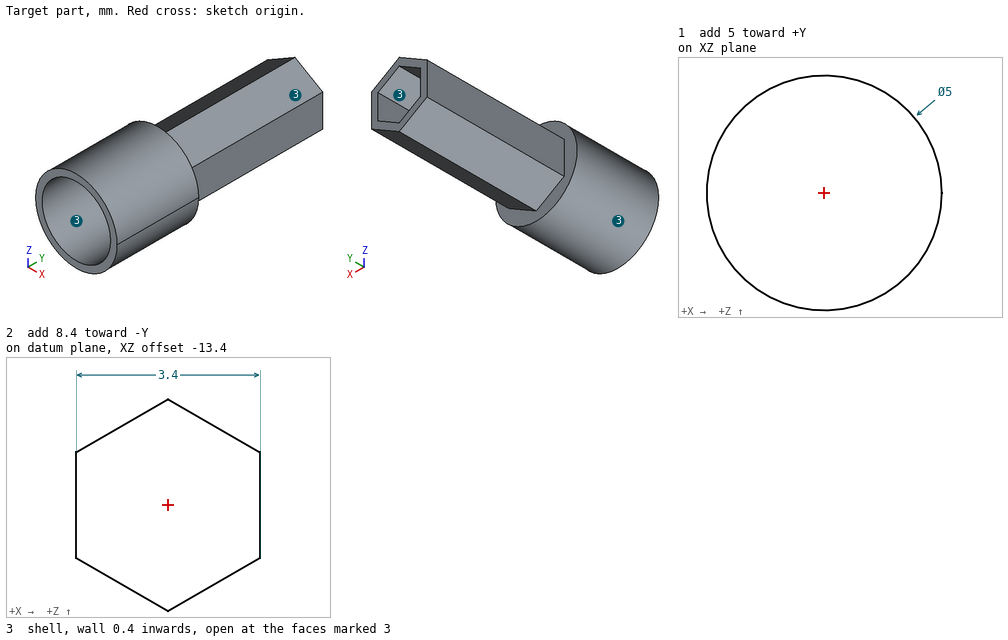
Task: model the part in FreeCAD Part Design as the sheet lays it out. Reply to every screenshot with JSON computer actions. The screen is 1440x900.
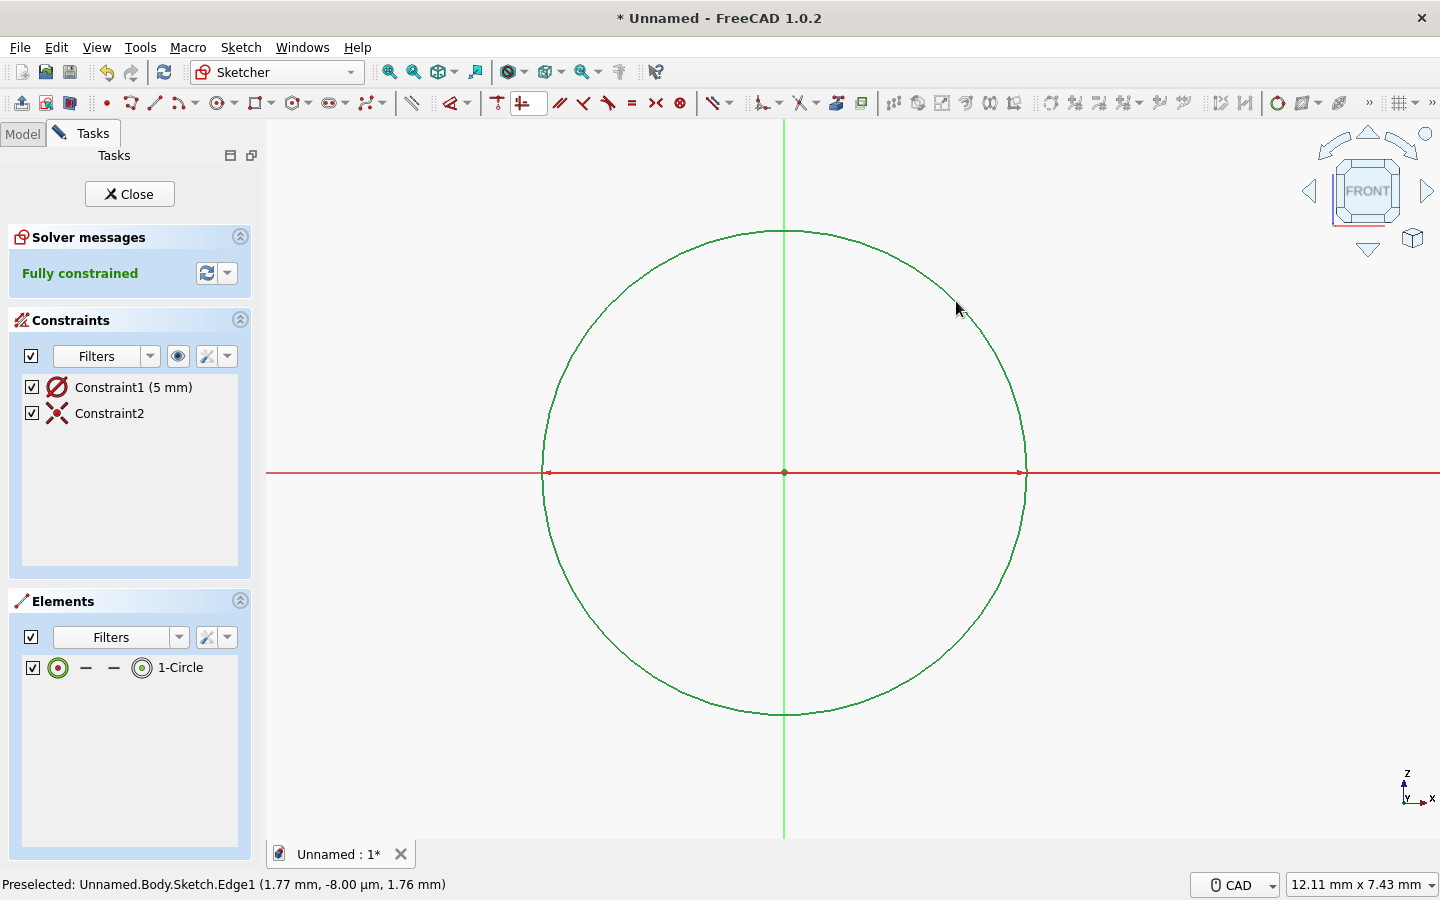
{"action": "left_click", "coordinate": [130, 194]}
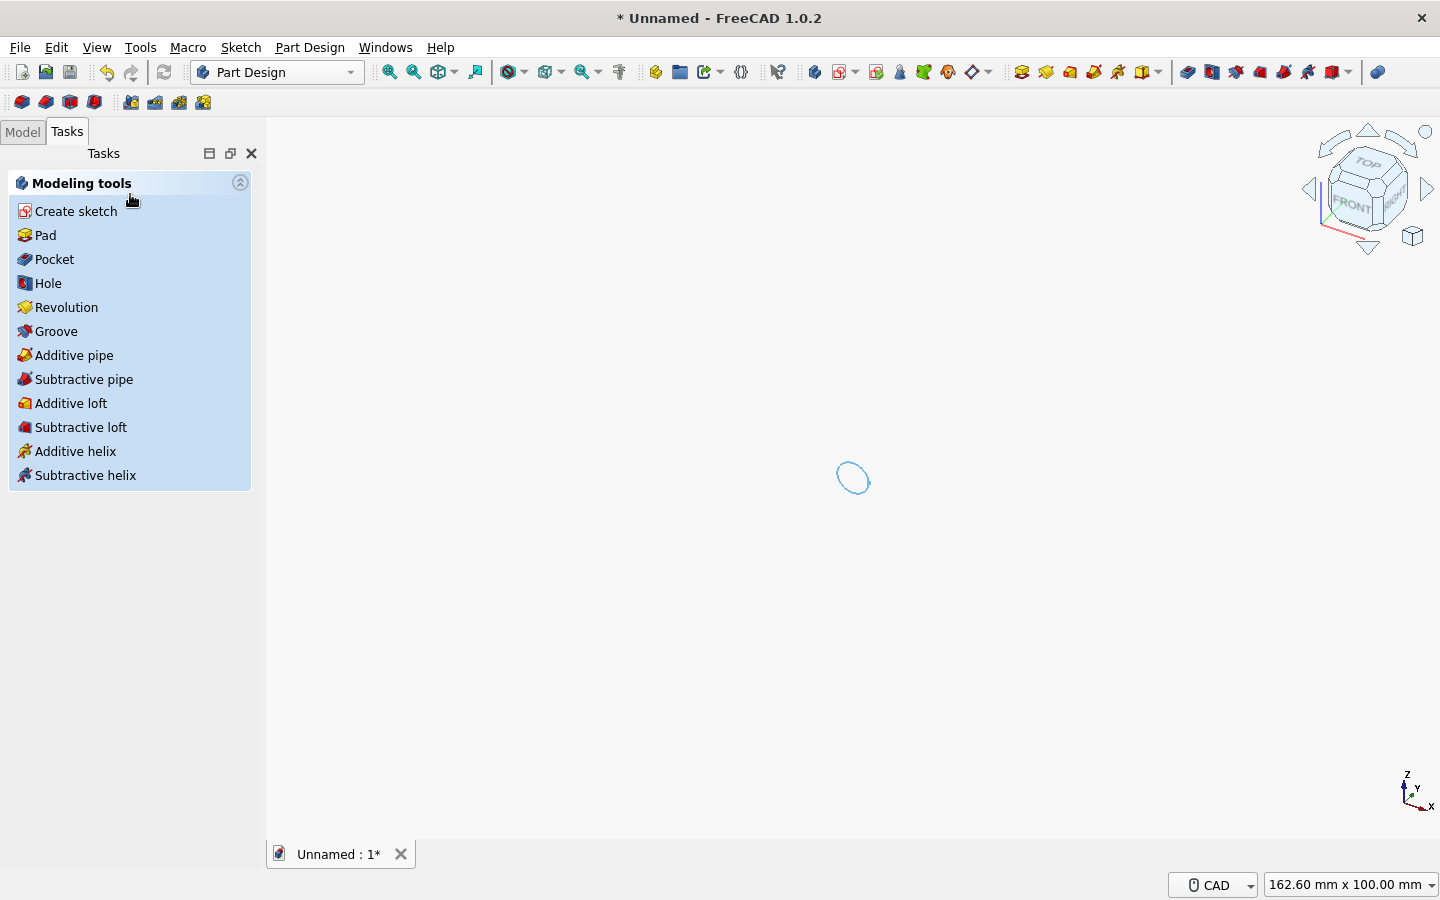
{"action": "left_click", "coordinate": [1022, 72]}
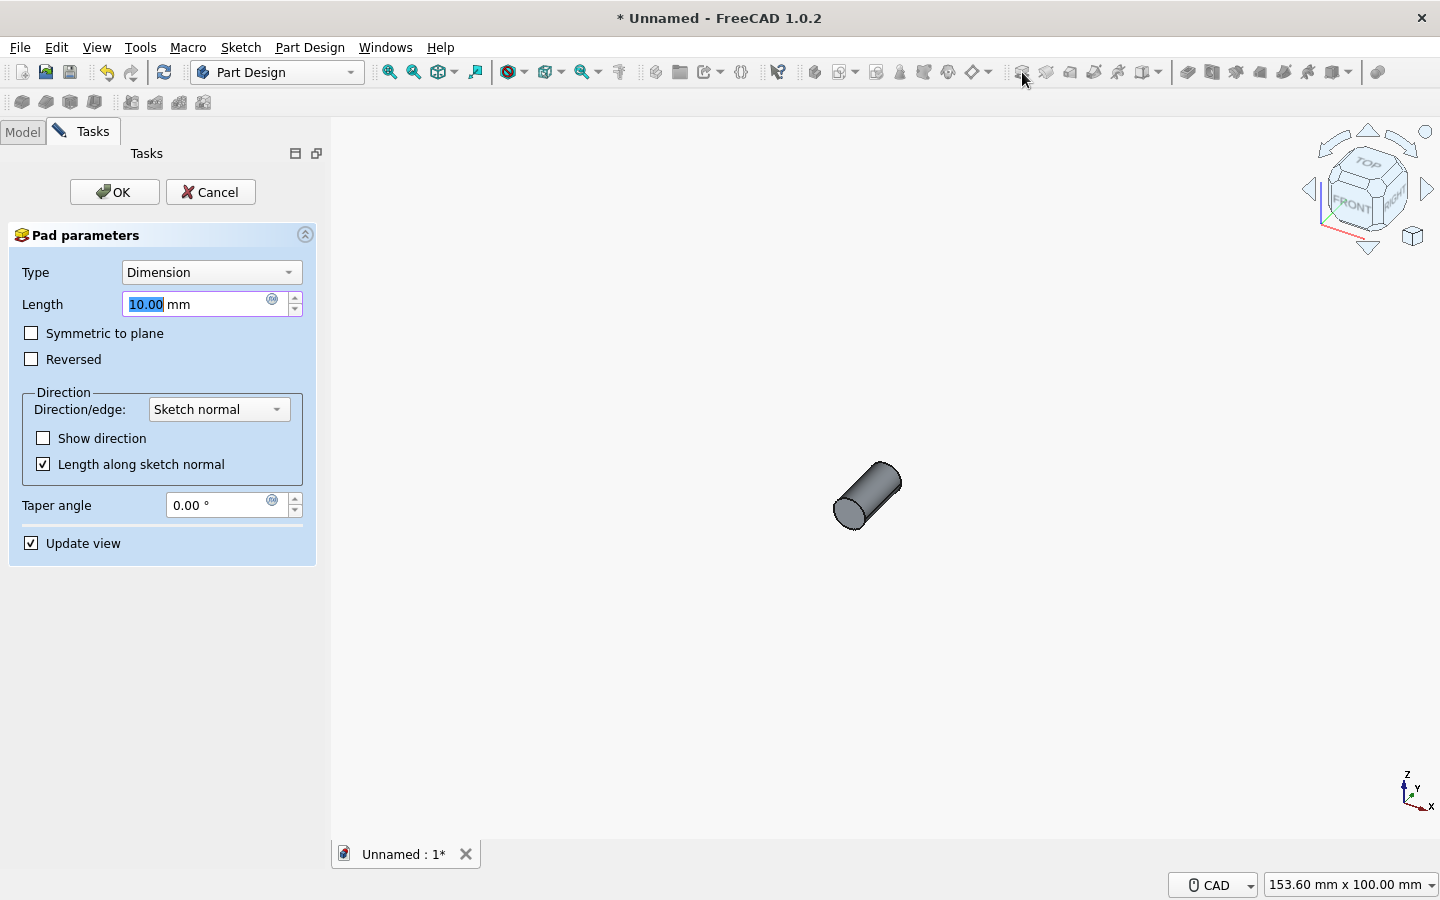
{"action": "type", "text": "5"}
{"action": "key", "text": "Tab"}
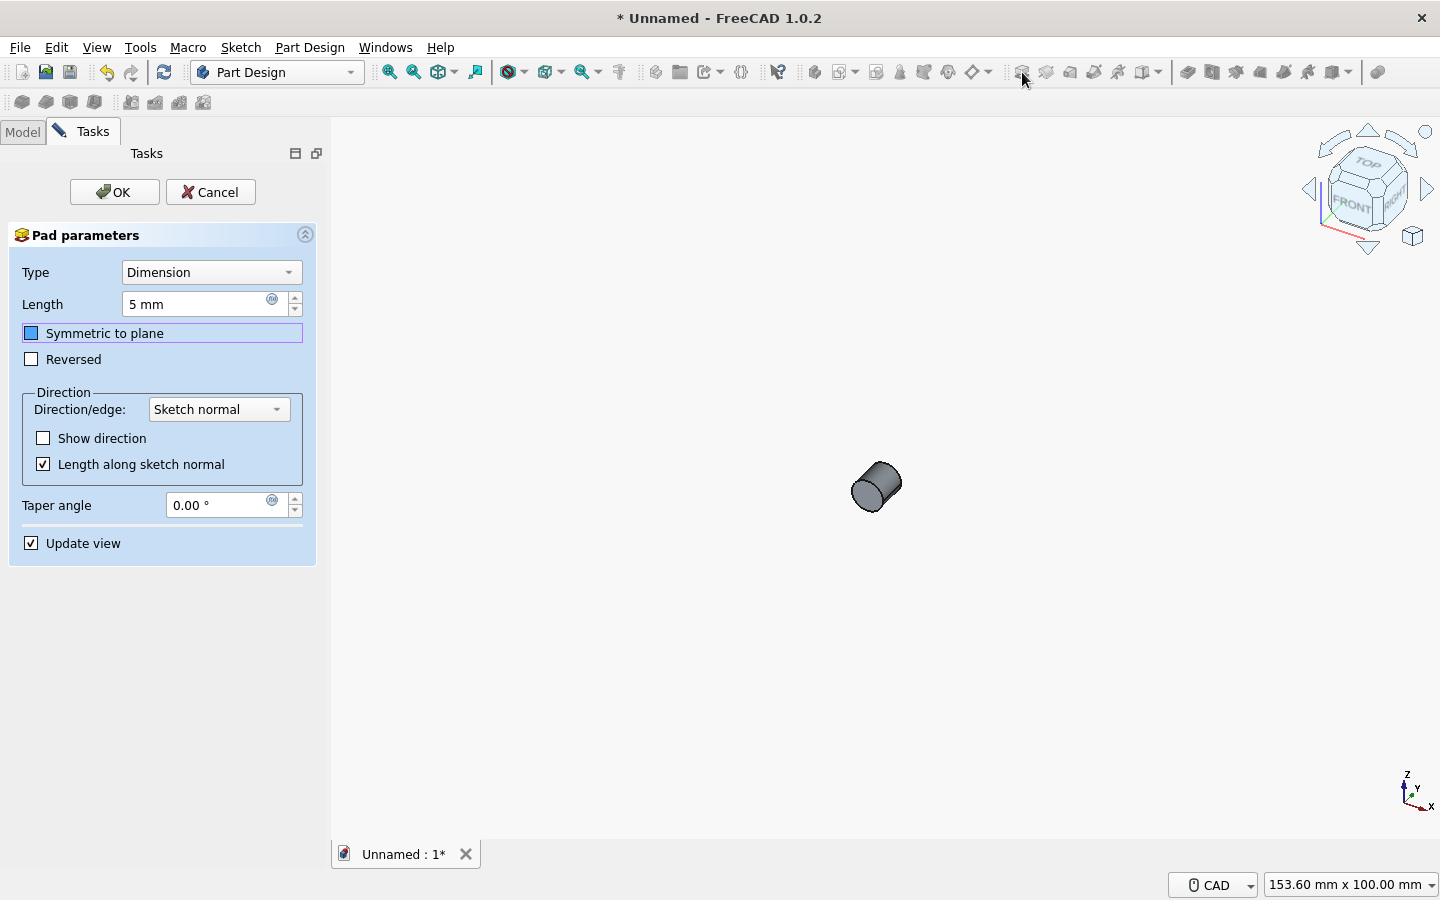
{"action": "left_click", "coordinate": [30, 359]}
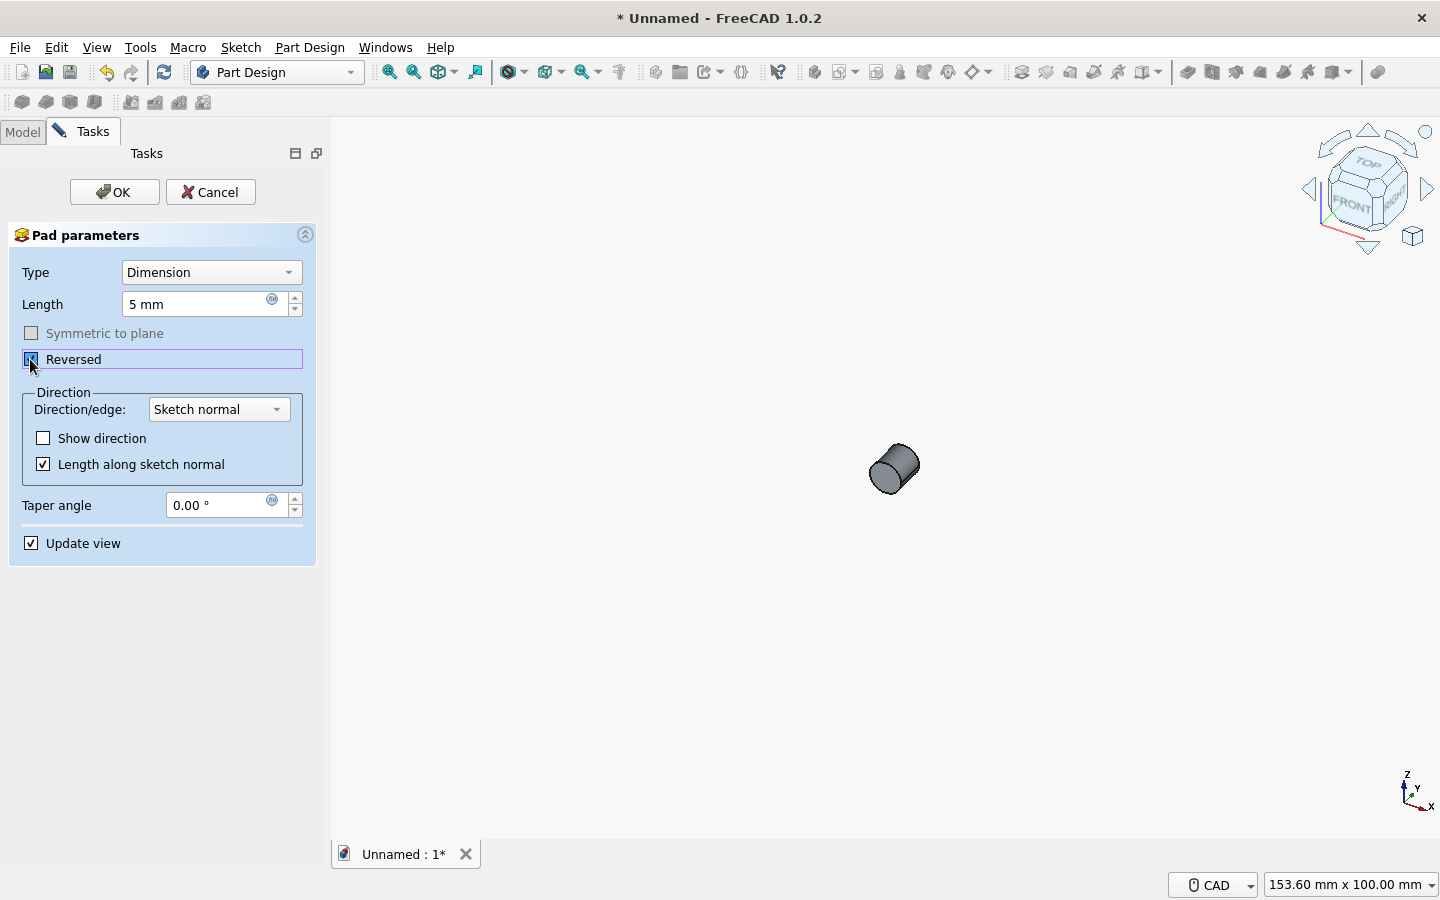
{"action": "left_click", "coordinate": [115, 192]}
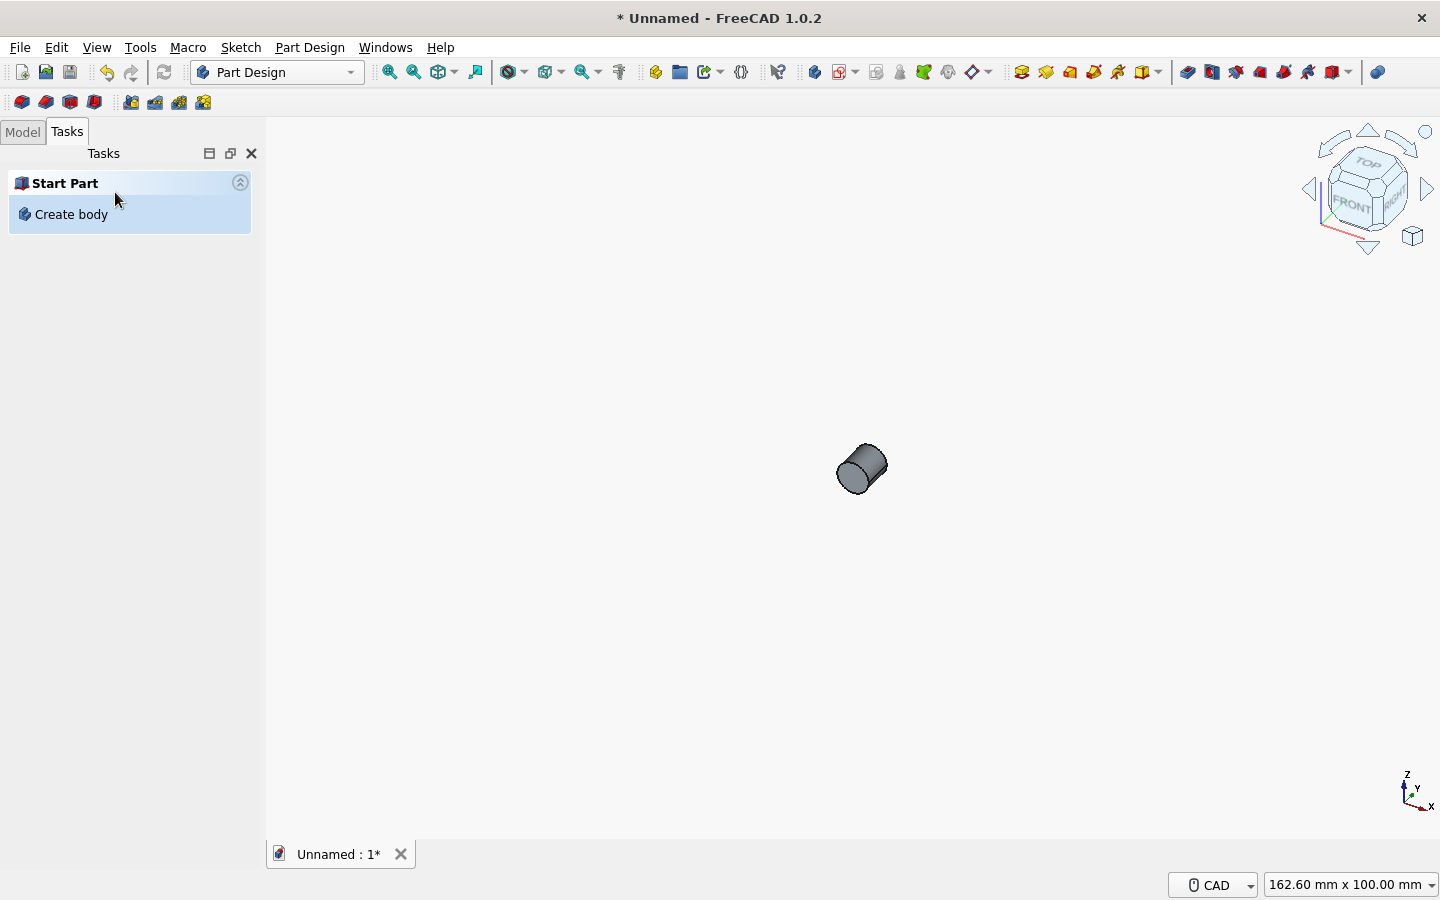
{"action": "left_click", "coordinate": [390, 72]}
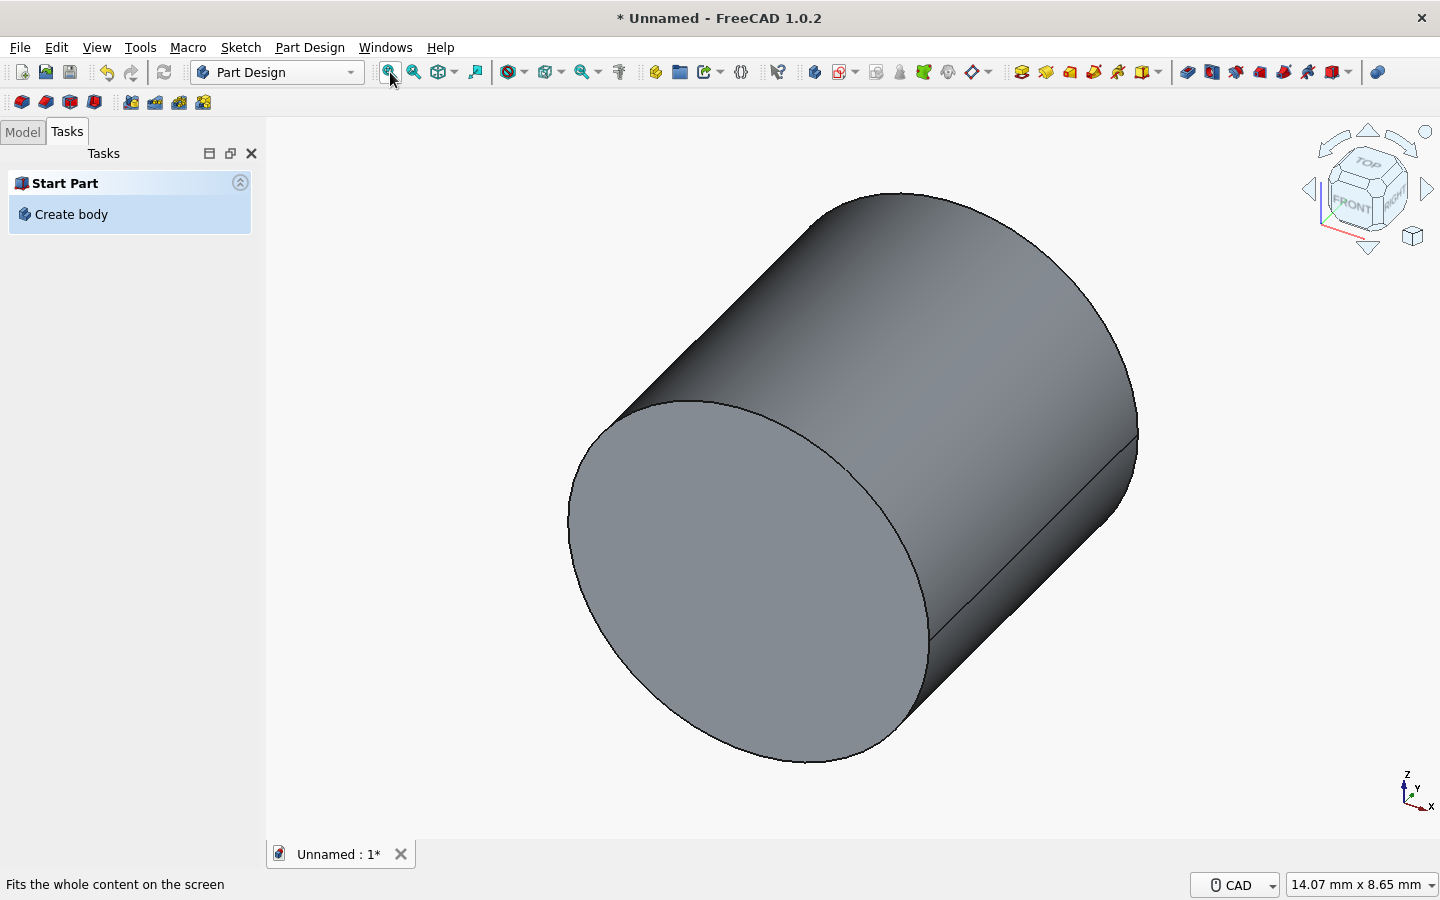
{"action": "left_click", "coordinate": [23, 131]}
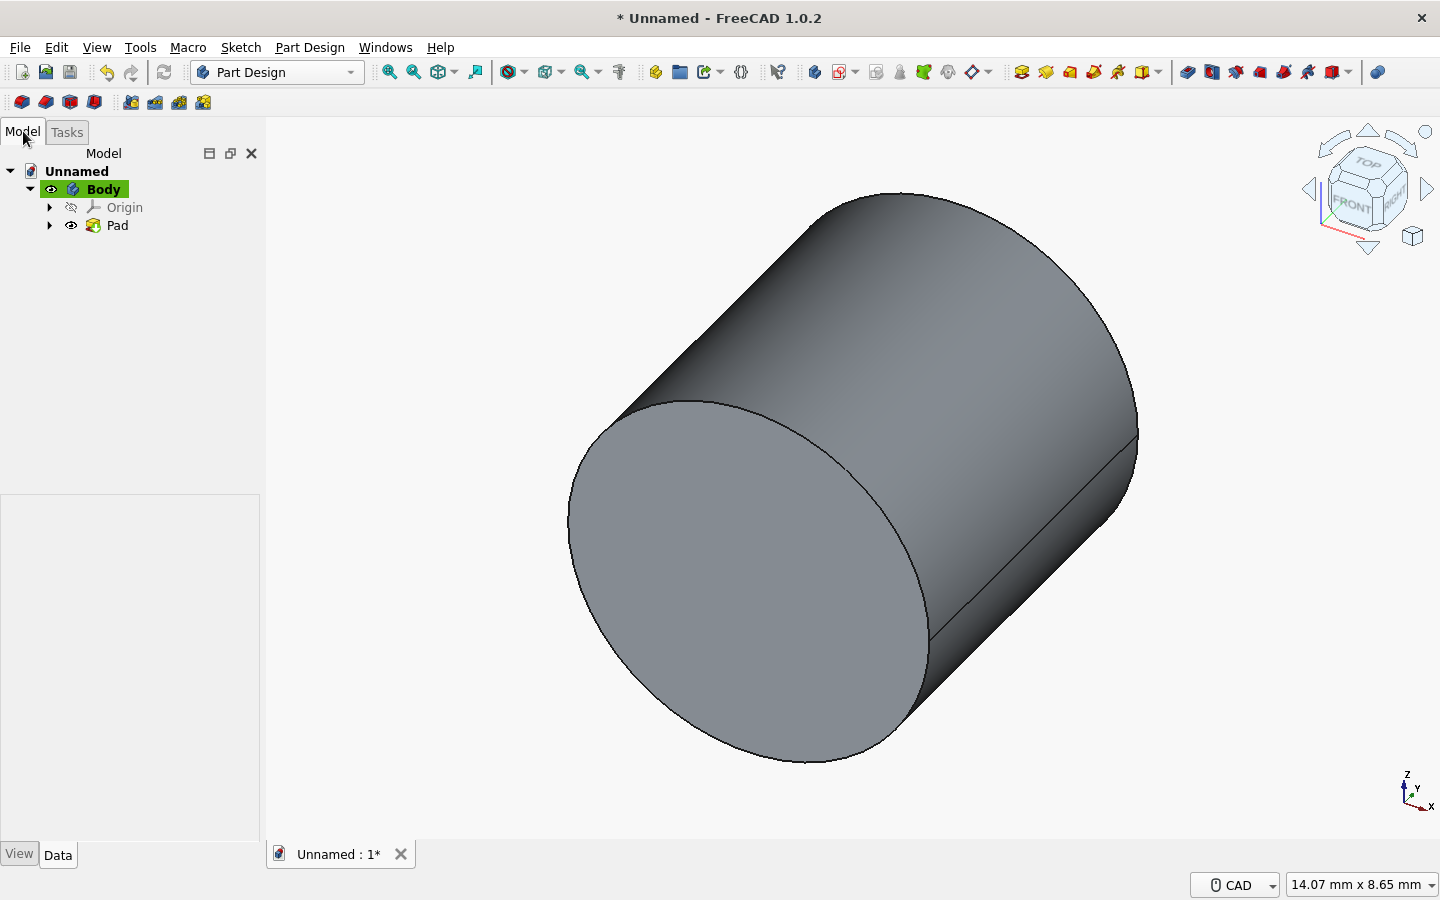
{"action": "left_click", "coordinate": [50, 207]}